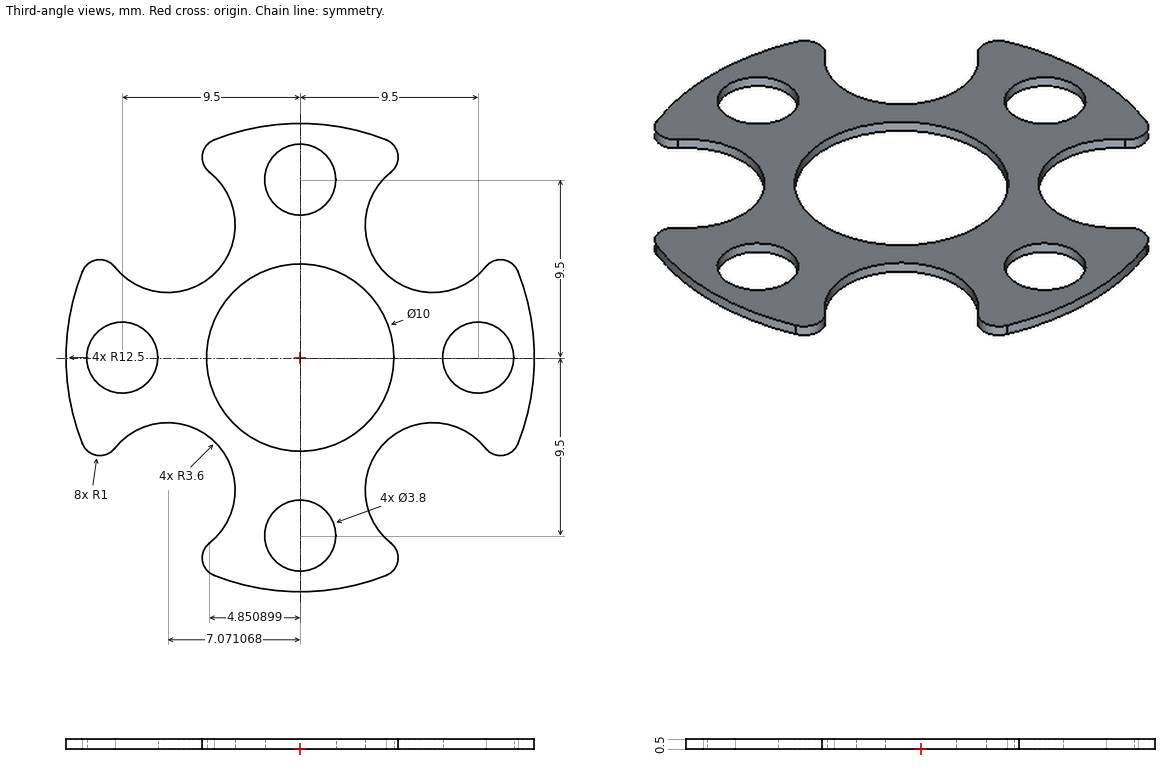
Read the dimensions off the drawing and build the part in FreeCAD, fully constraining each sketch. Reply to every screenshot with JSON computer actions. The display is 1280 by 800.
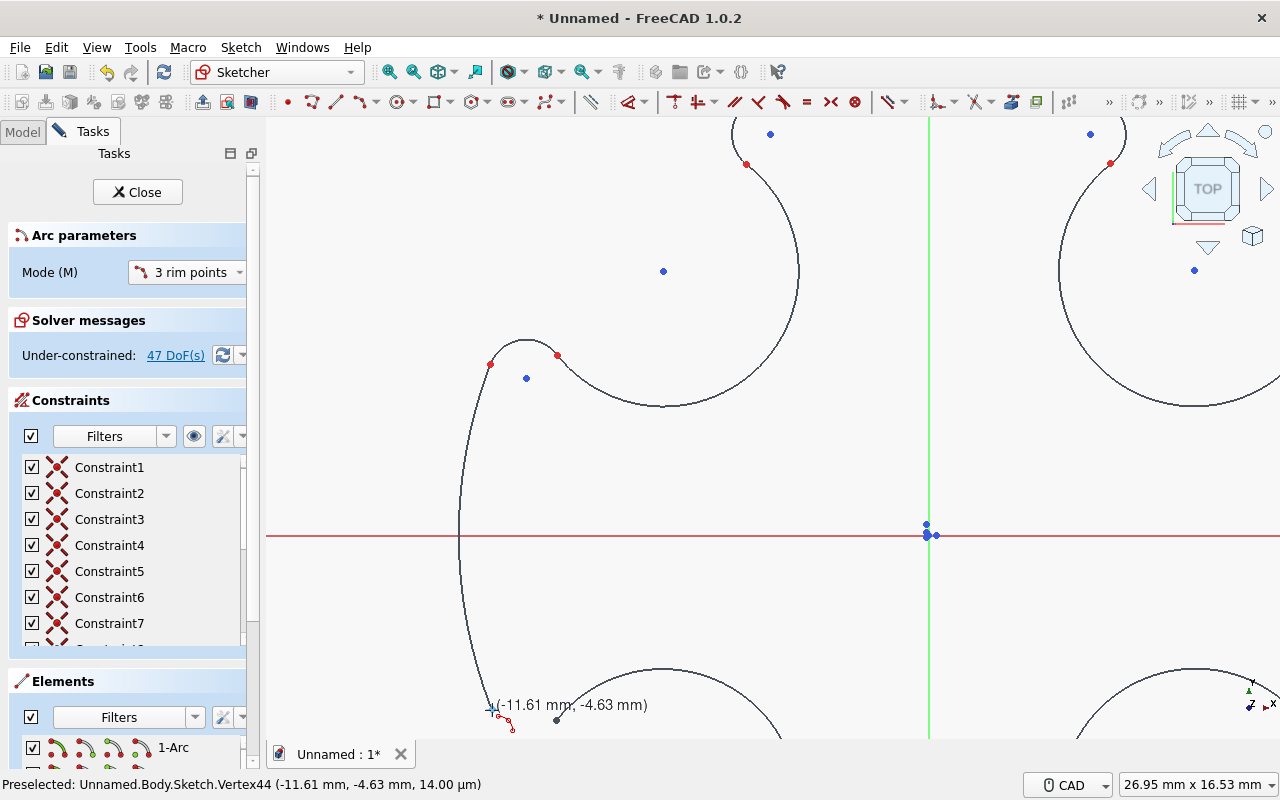
{"action": "scroll", "coordinate": [521, 340], "scroll_direction": "down", "scroll_amount": 4}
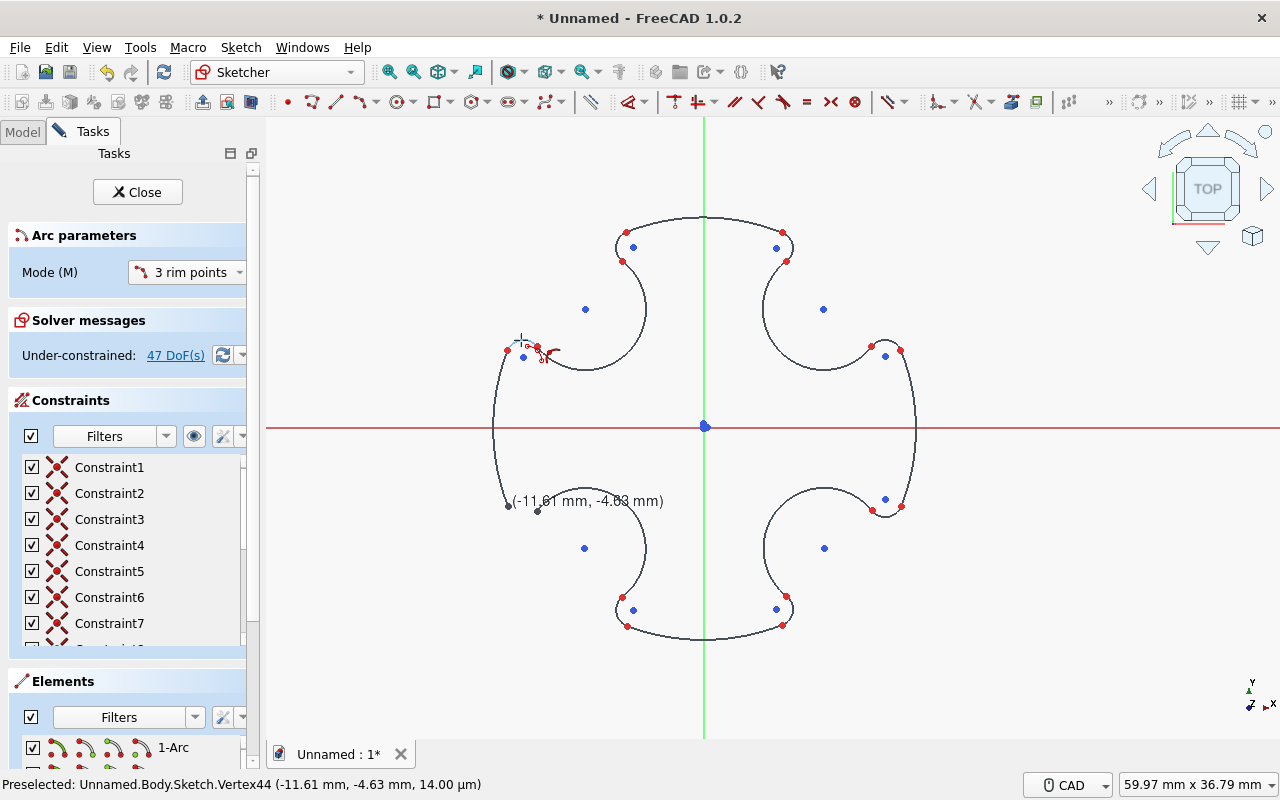
{"action": "left_click", "coordinate": [537, 511]}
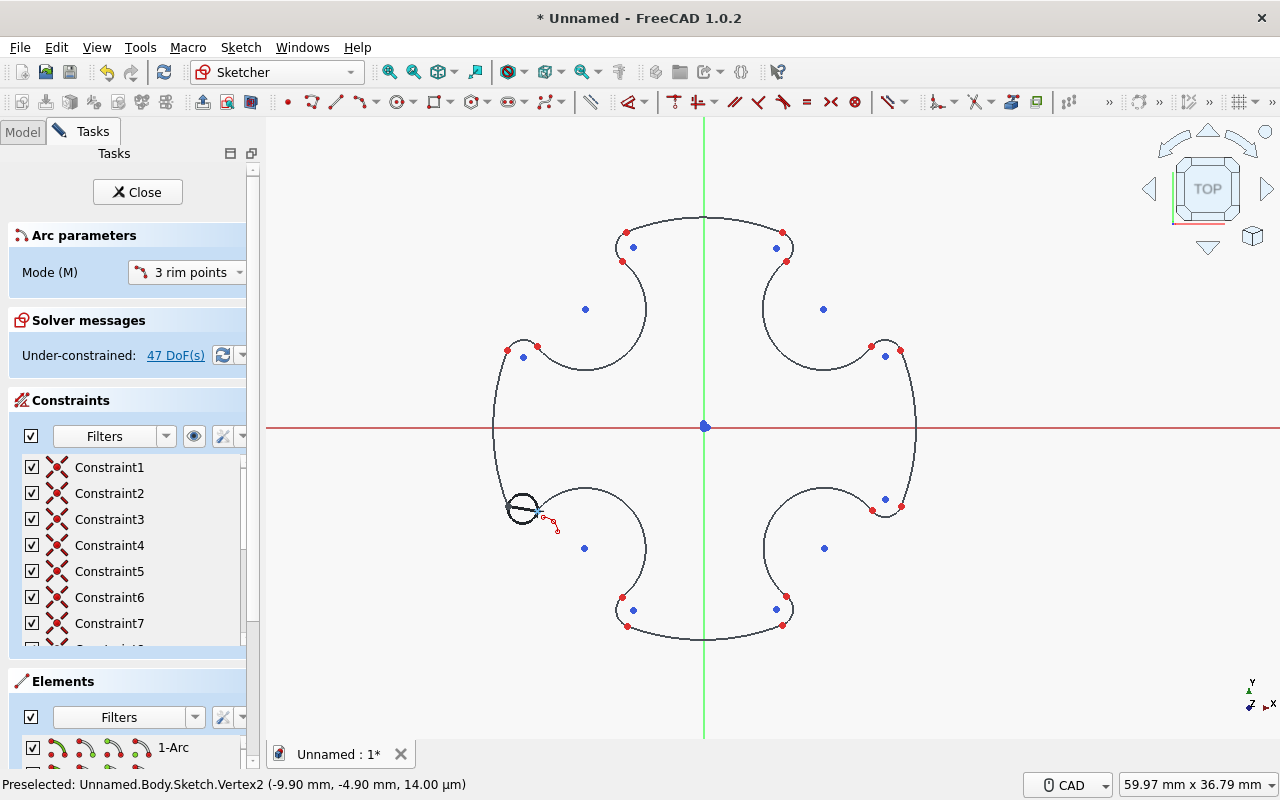
{"action": "scroll", "coordinate": [521, 517], "scroll_direction": "up", "scroll_amount": 4}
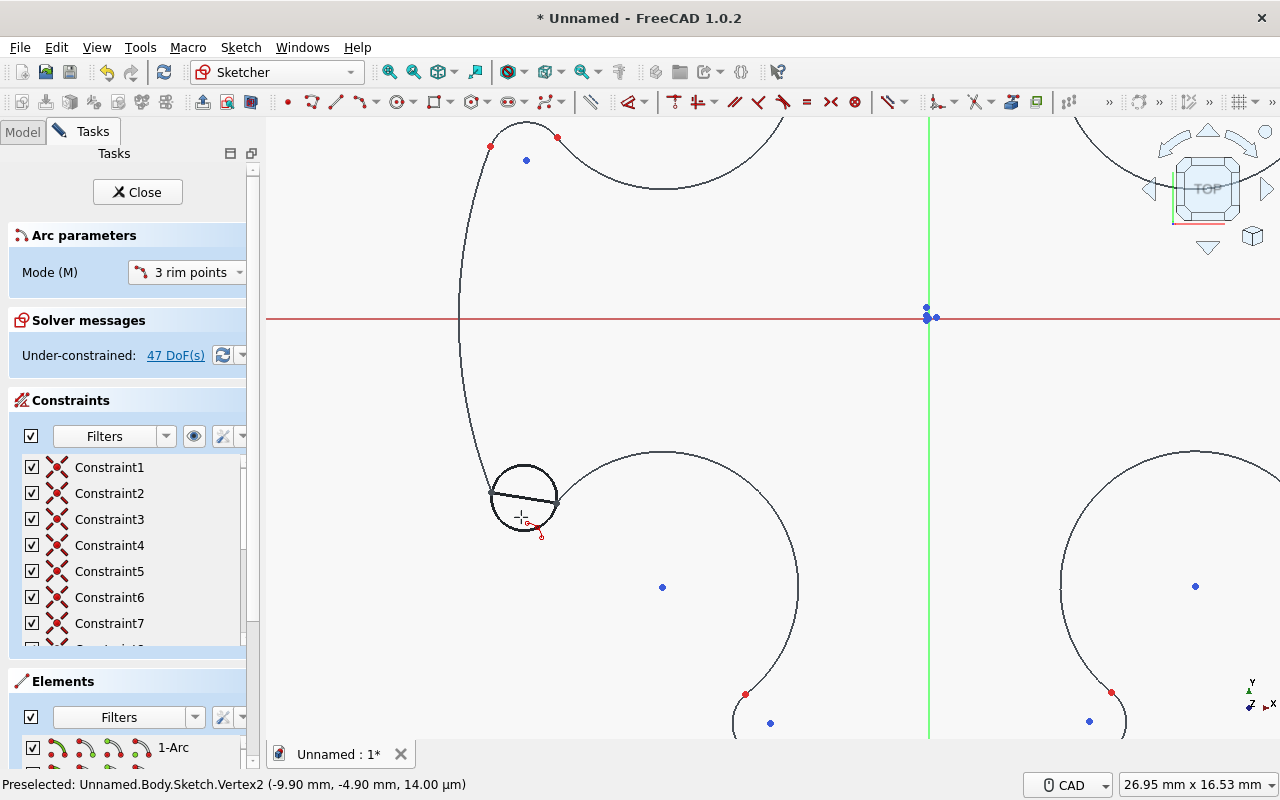
{"action": "left_click", "coordinate": [521, 515]}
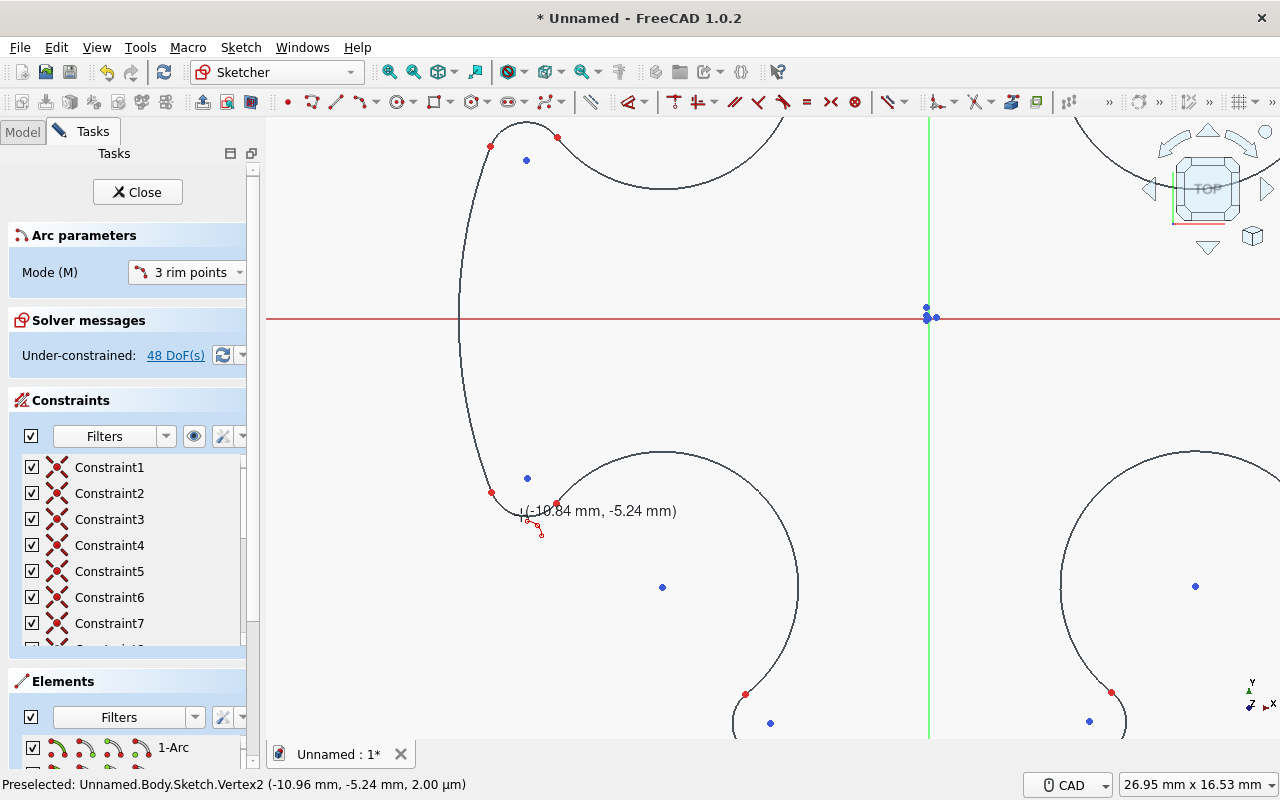
{"action": "key", "text": "g c"}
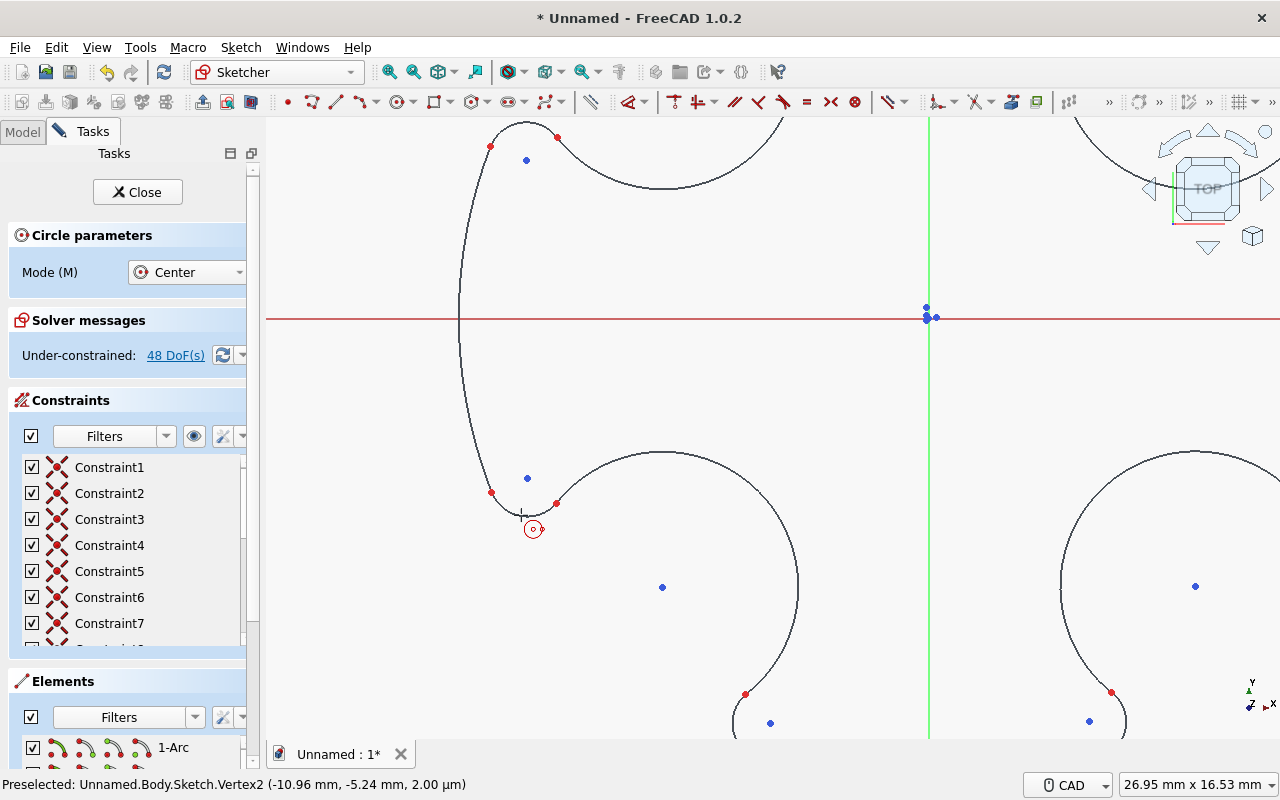
{"action": "left_click", "coordinate": [929, 676]}
{"action": "left_click", "coordinate": [980, 626]}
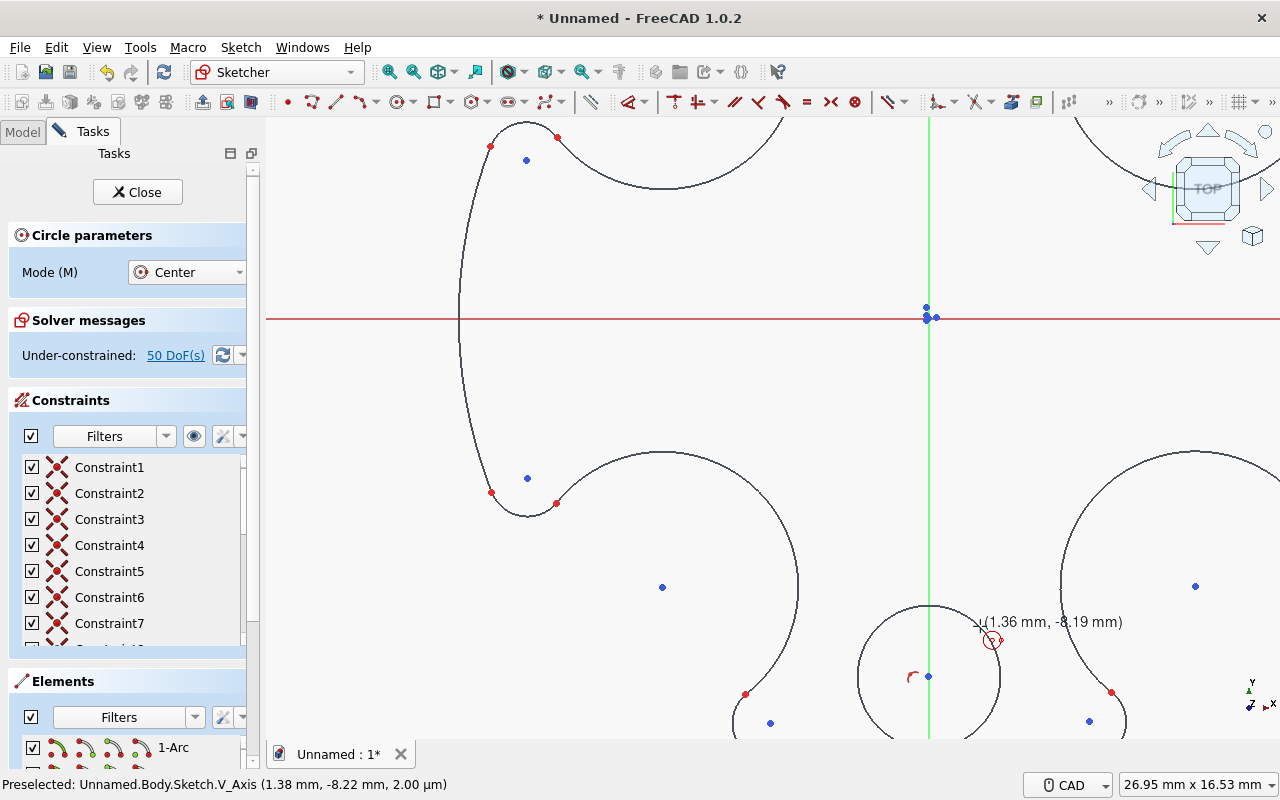
{"action": "left_click", "coordinate": [571, 319]}
{"action": "left_click", "coordinate": [622, 268]}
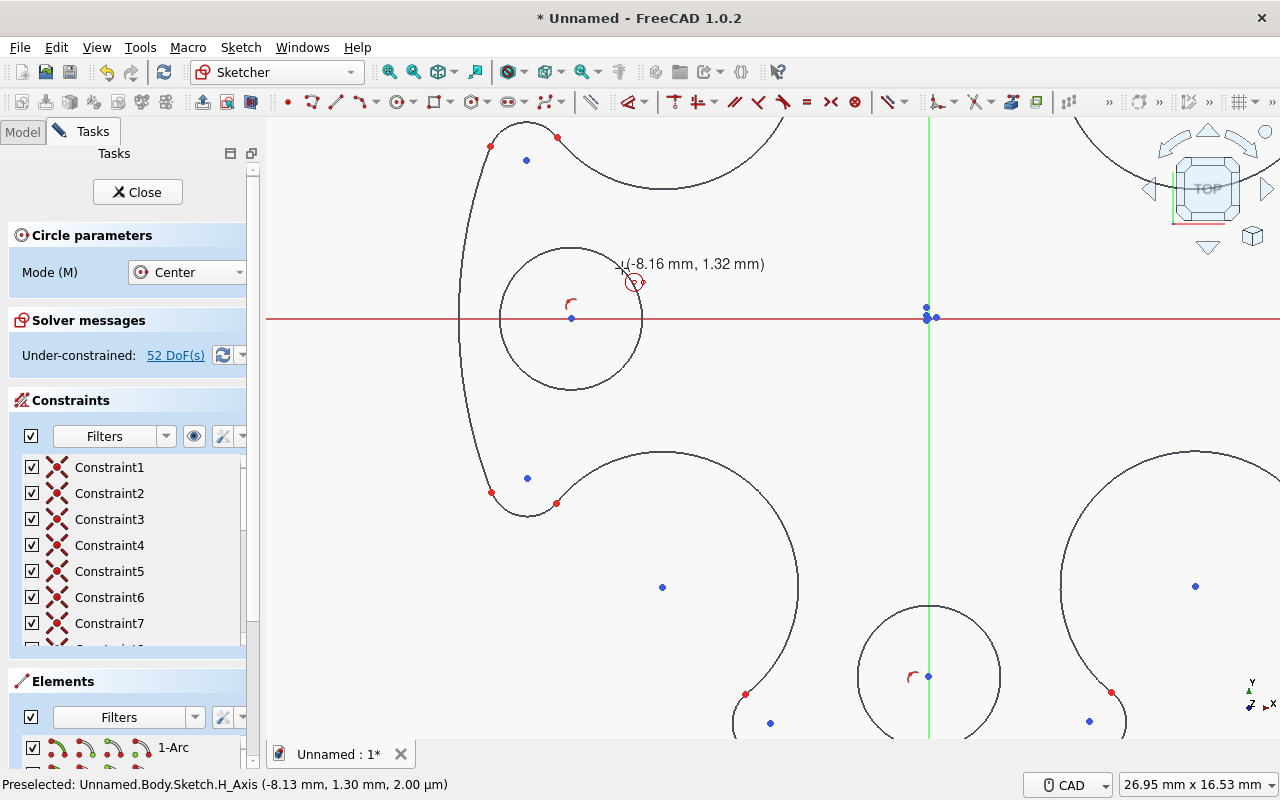
{"action": "left_click", "coordinate": [929, 319]}
{"action": "left_click", "coordinate": [1062, 186]}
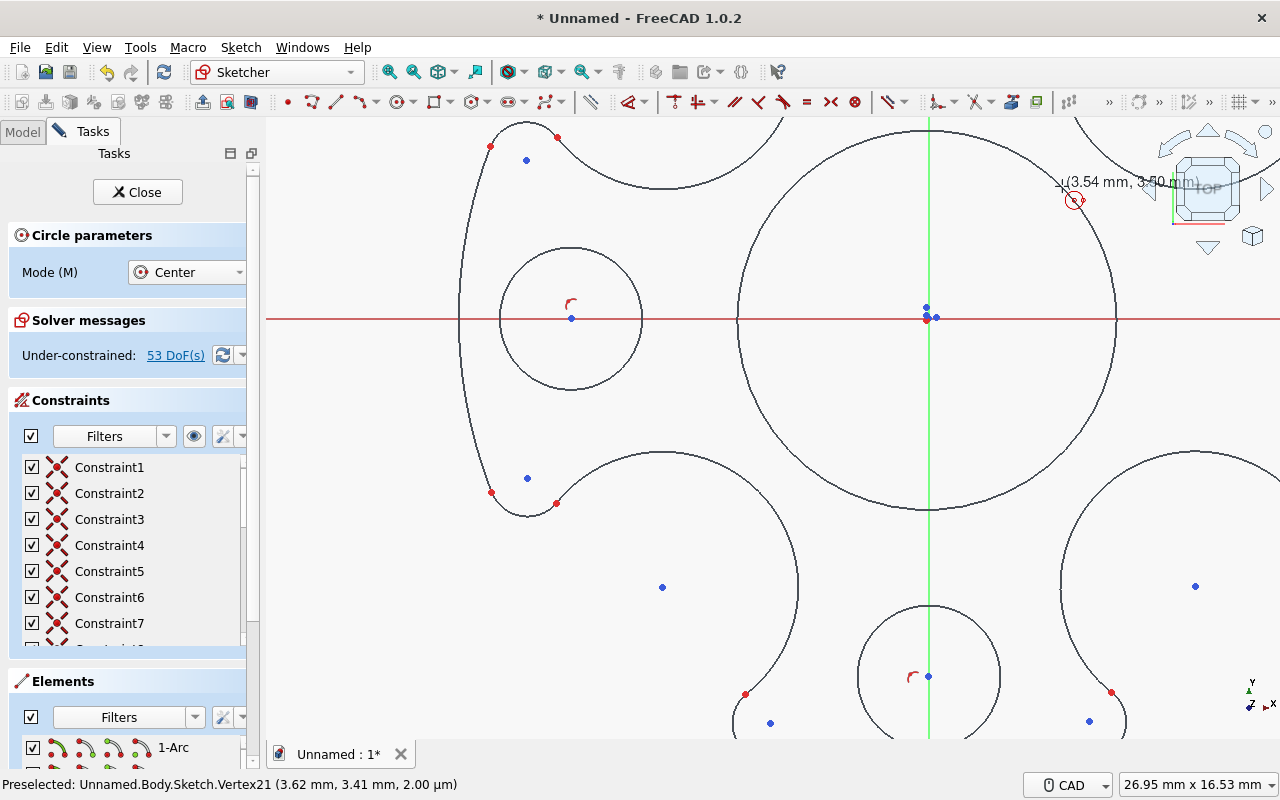
{"action": "scroll", "coordinate": [521, 517], "scroll_direction": "down", "scroll_amount": 4}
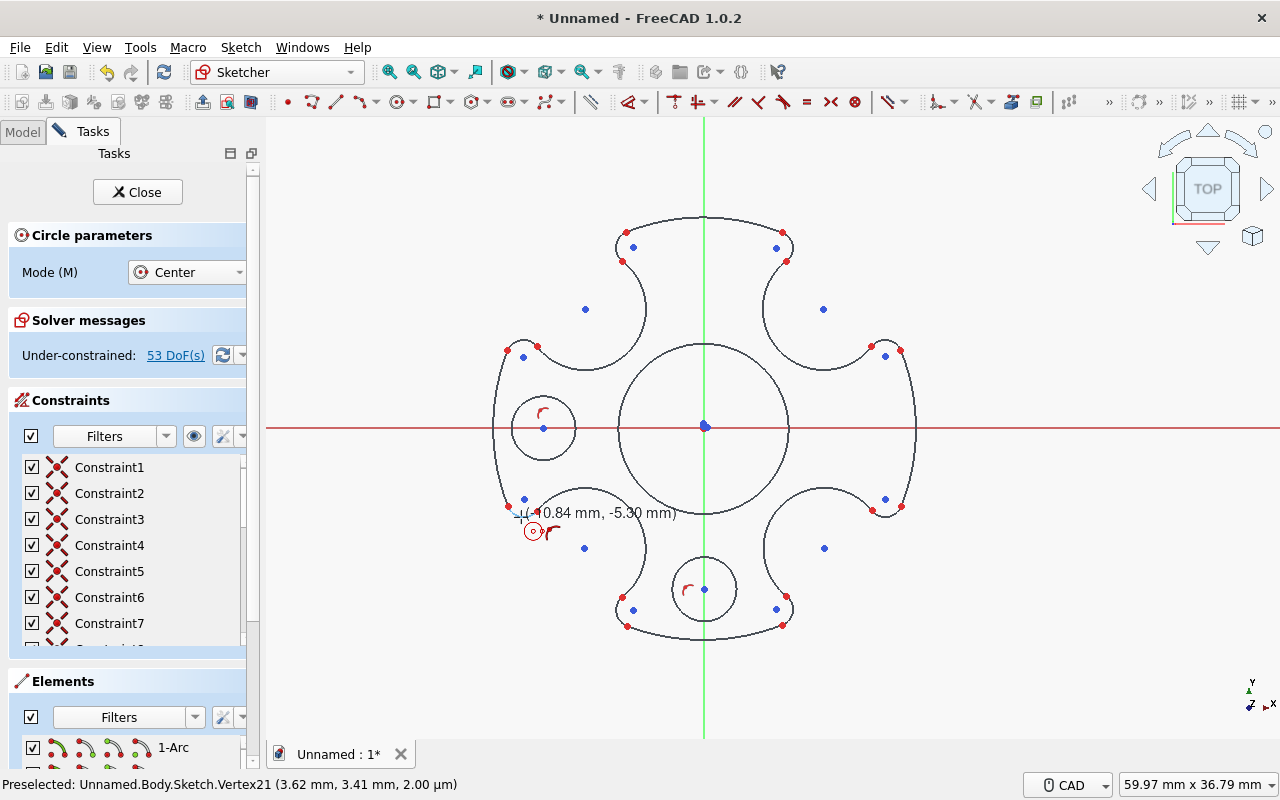
{"action": "left_click", "coordinate": [865, 428]}
{"action": "left_click", "coordinate": [888, 406]}